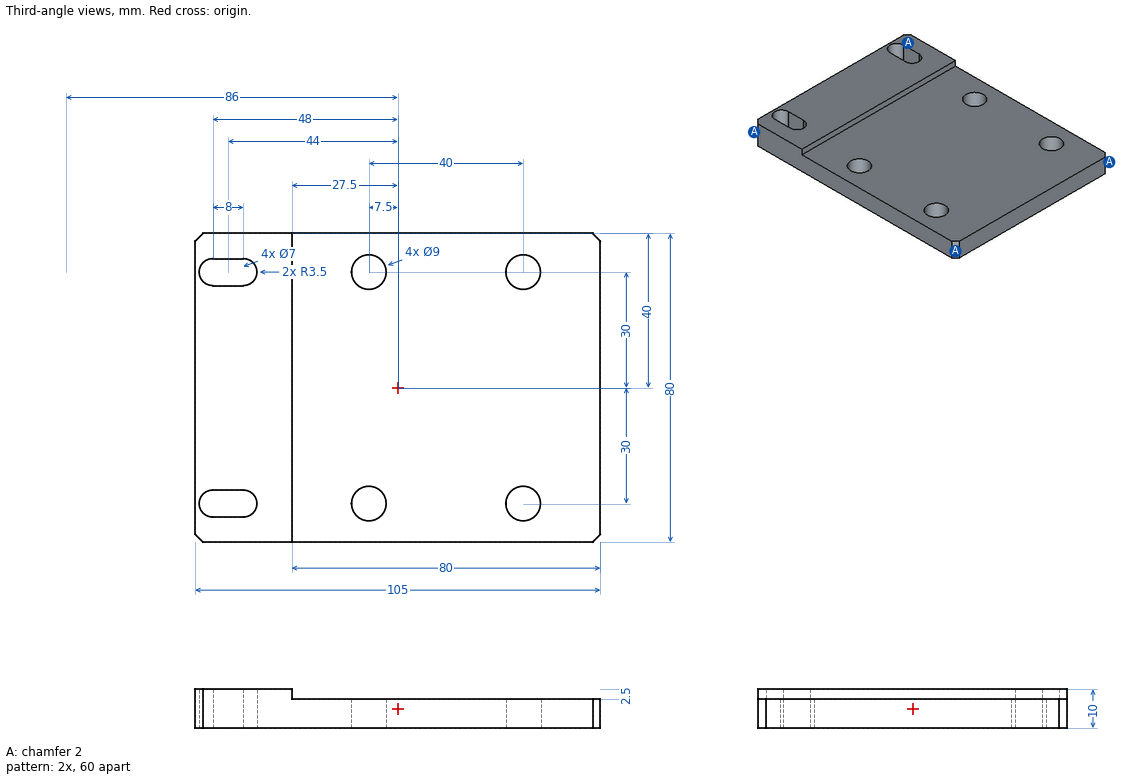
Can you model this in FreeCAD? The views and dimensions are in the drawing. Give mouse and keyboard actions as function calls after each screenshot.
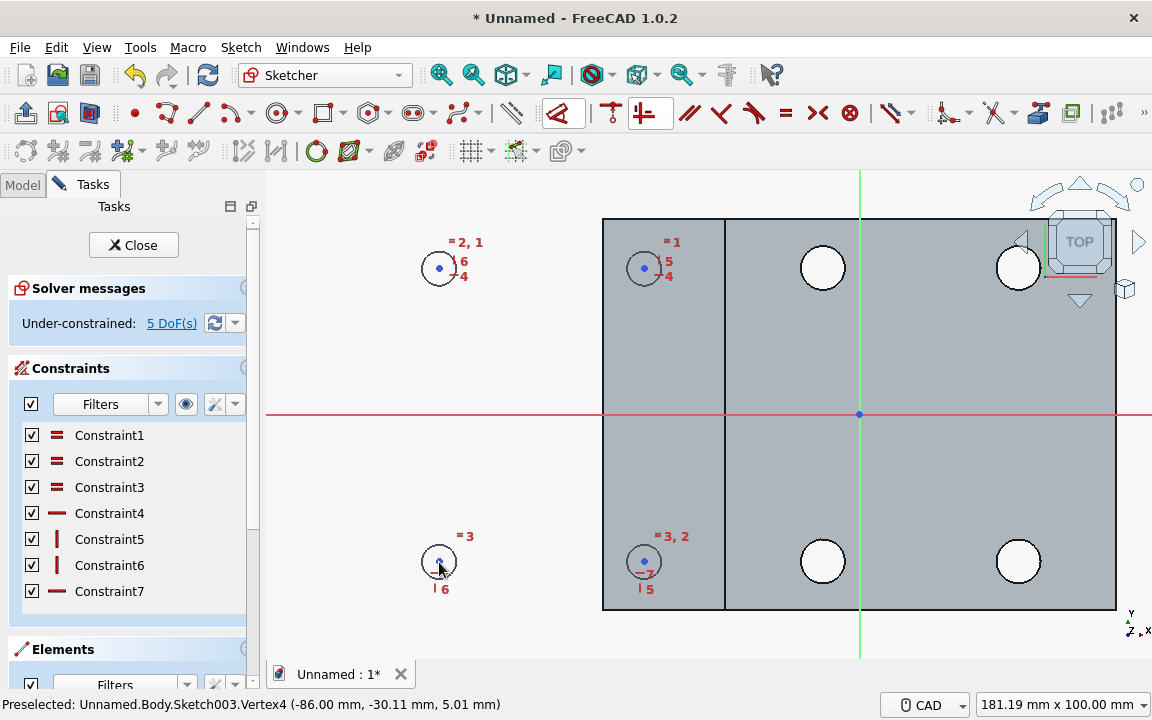
click(632, 257)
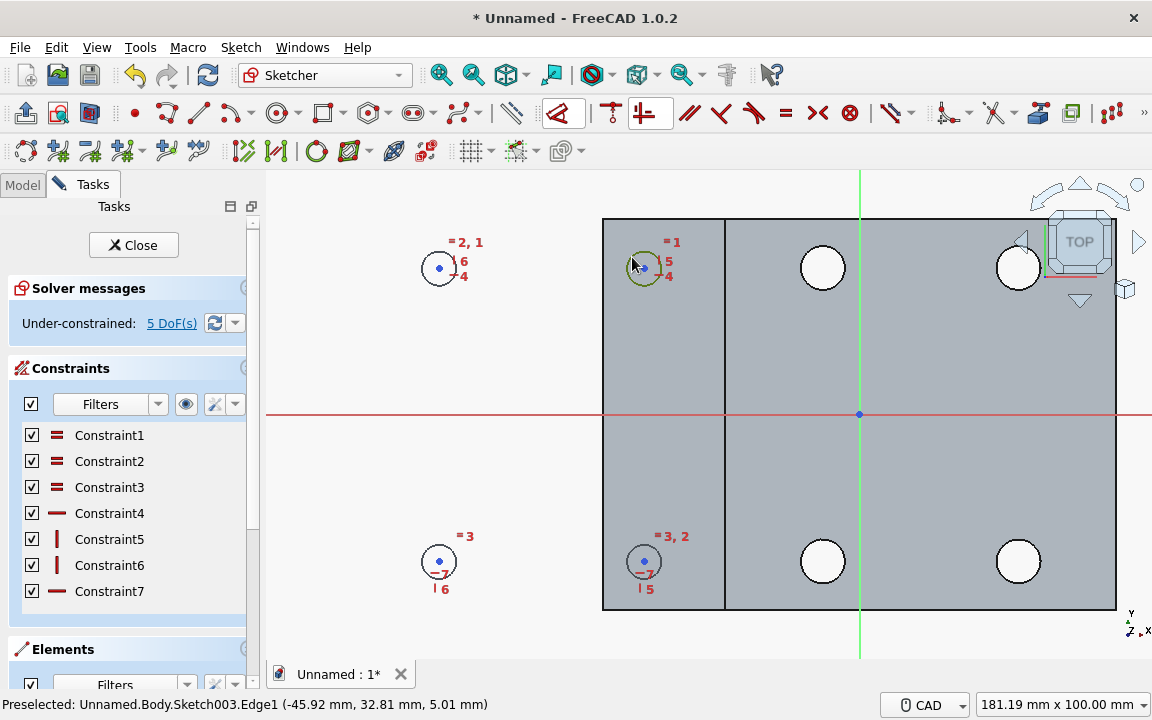
click(580, 114)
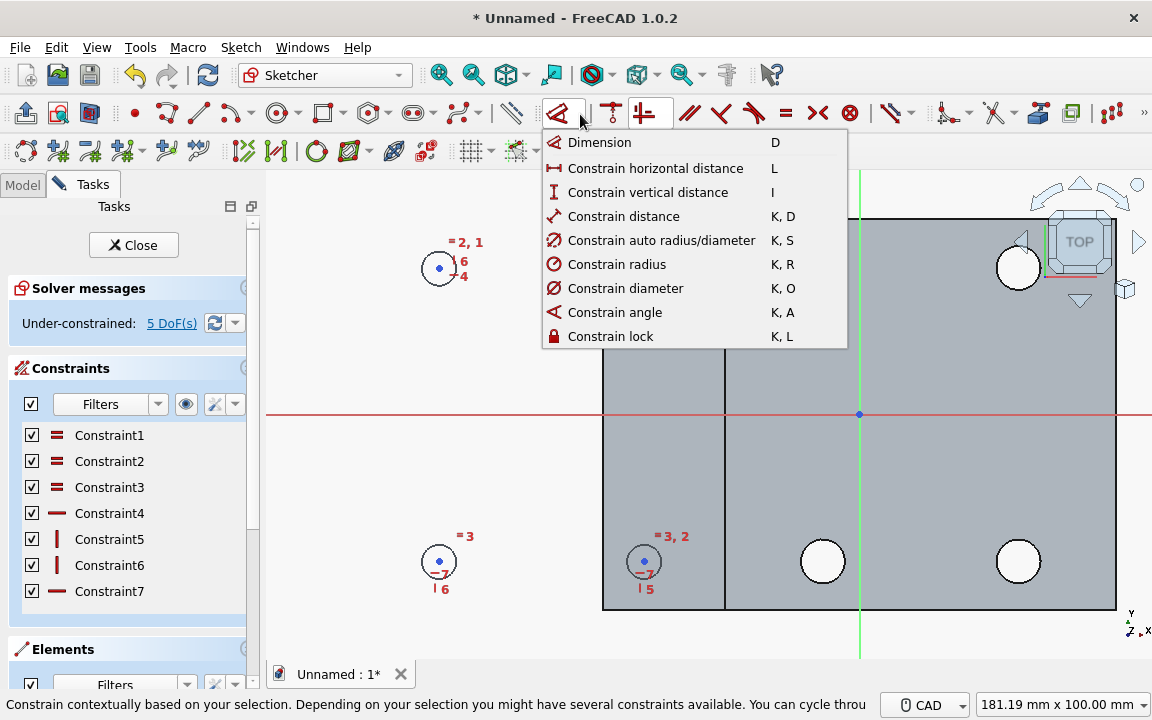
click(695, 288)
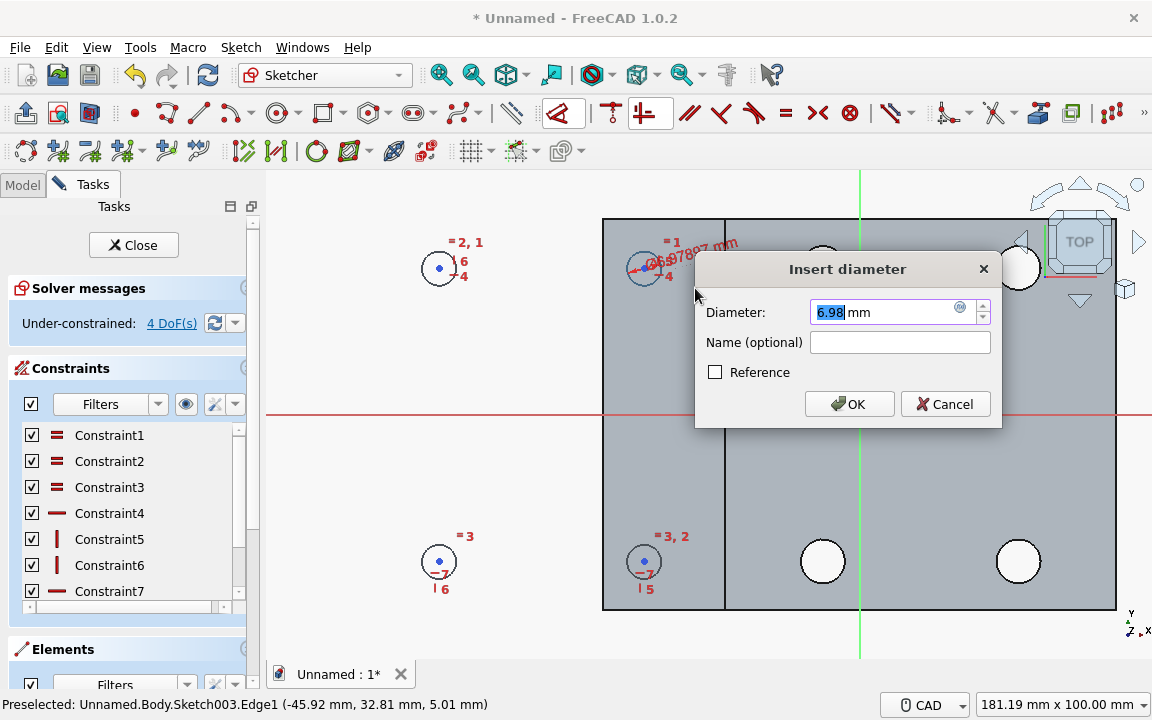
text(7)
key(Return)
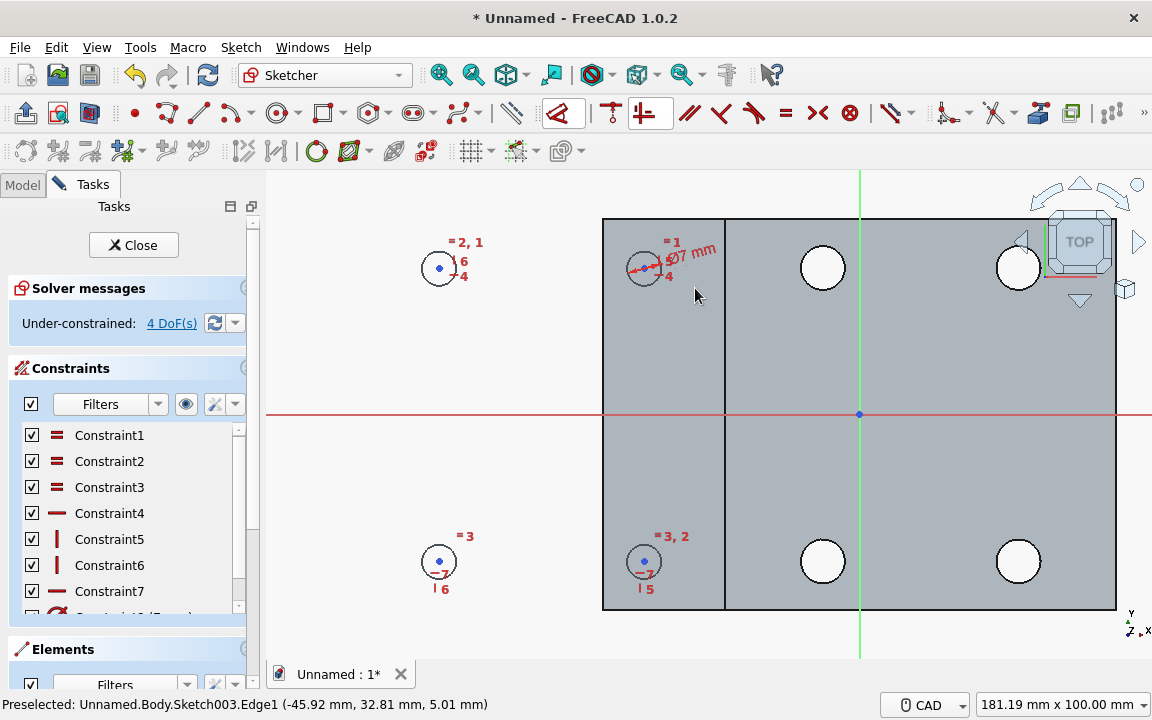
click(644, 269)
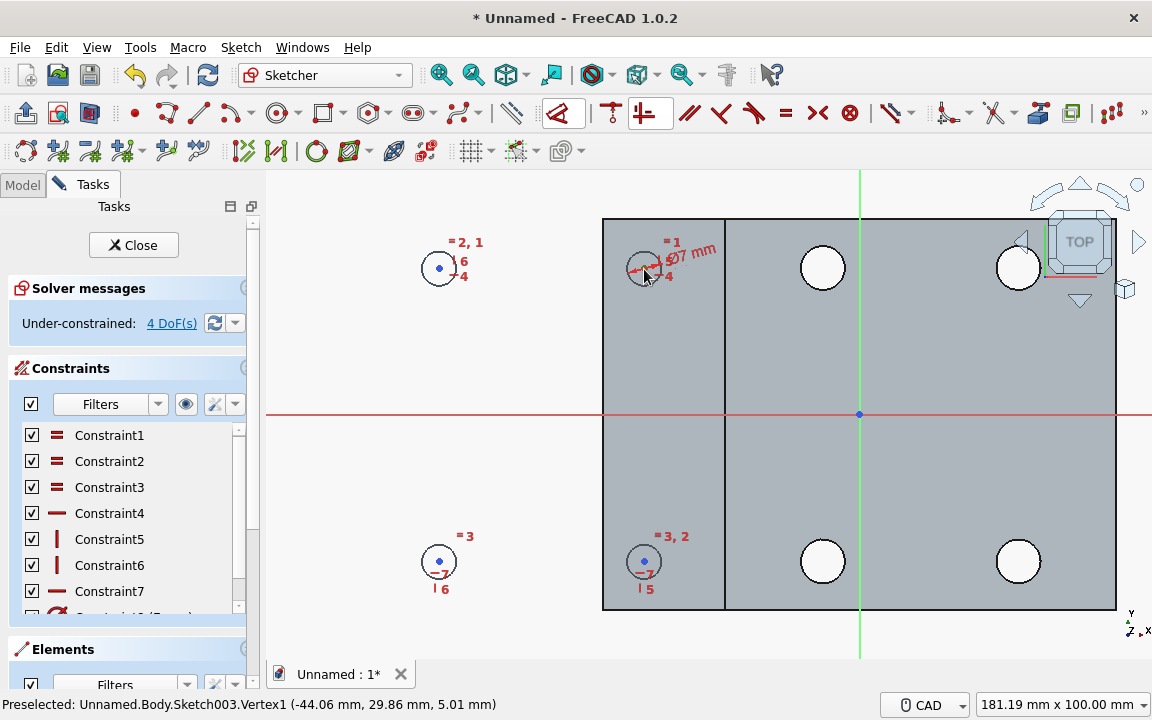
click(580, 114)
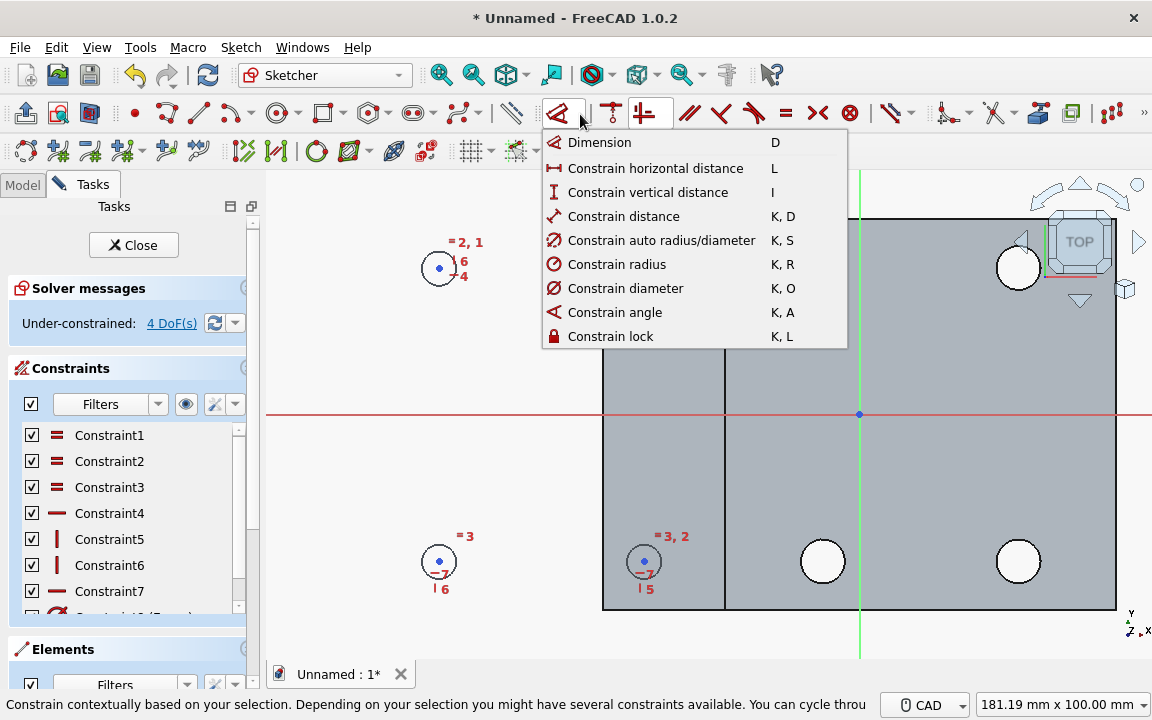
click(695, 168)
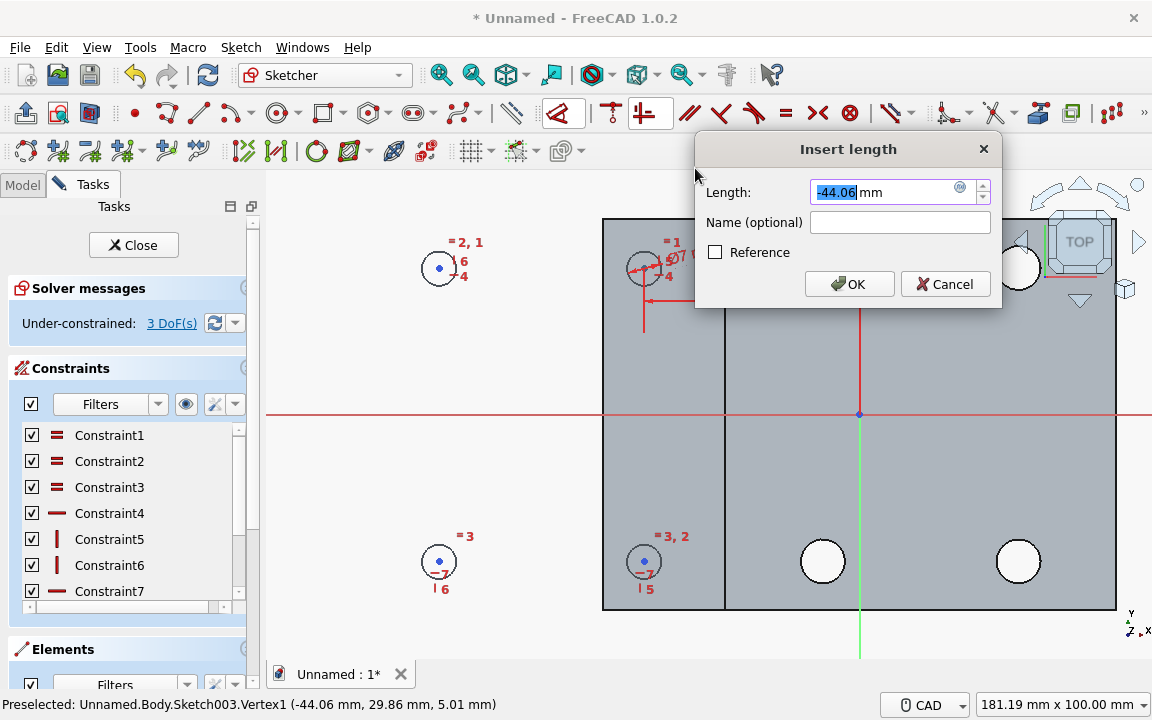
text(-44)
key(Return)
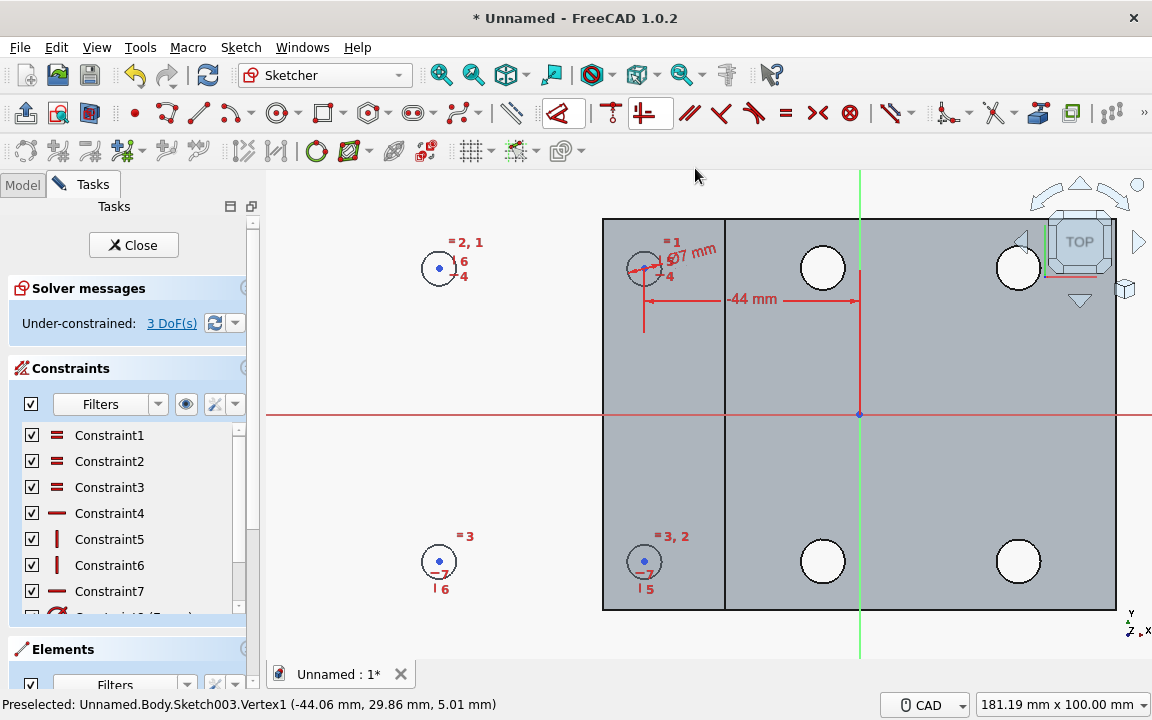
click(644, 269)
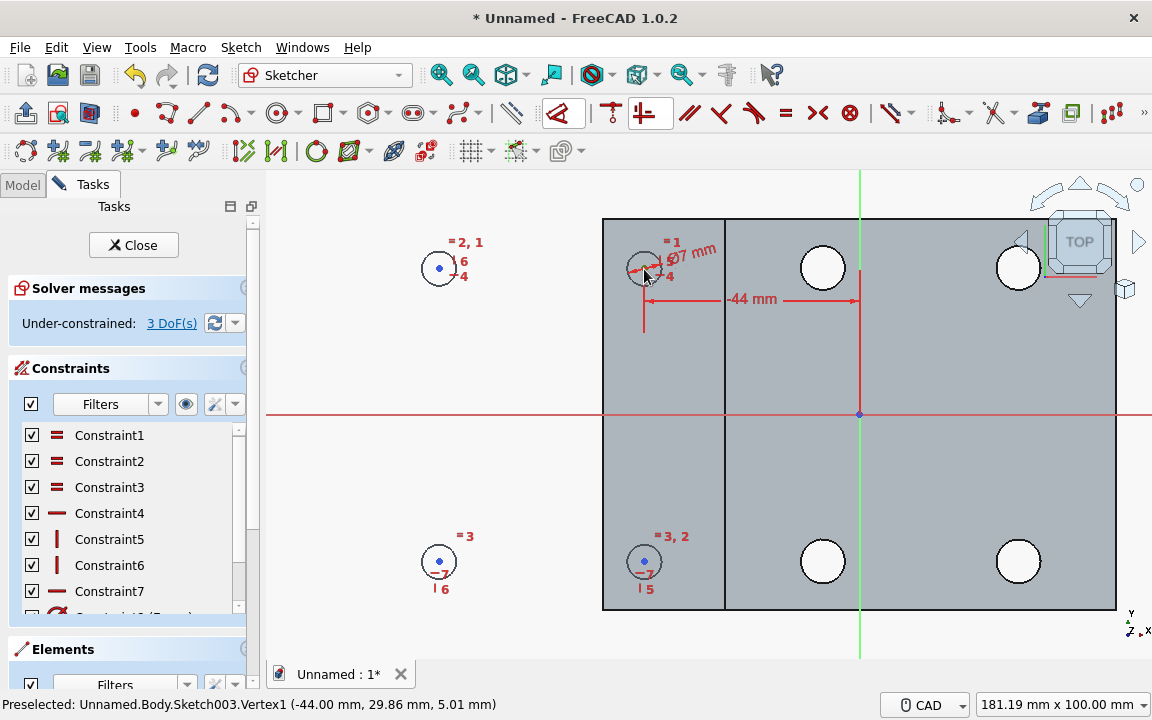
click(580, 114)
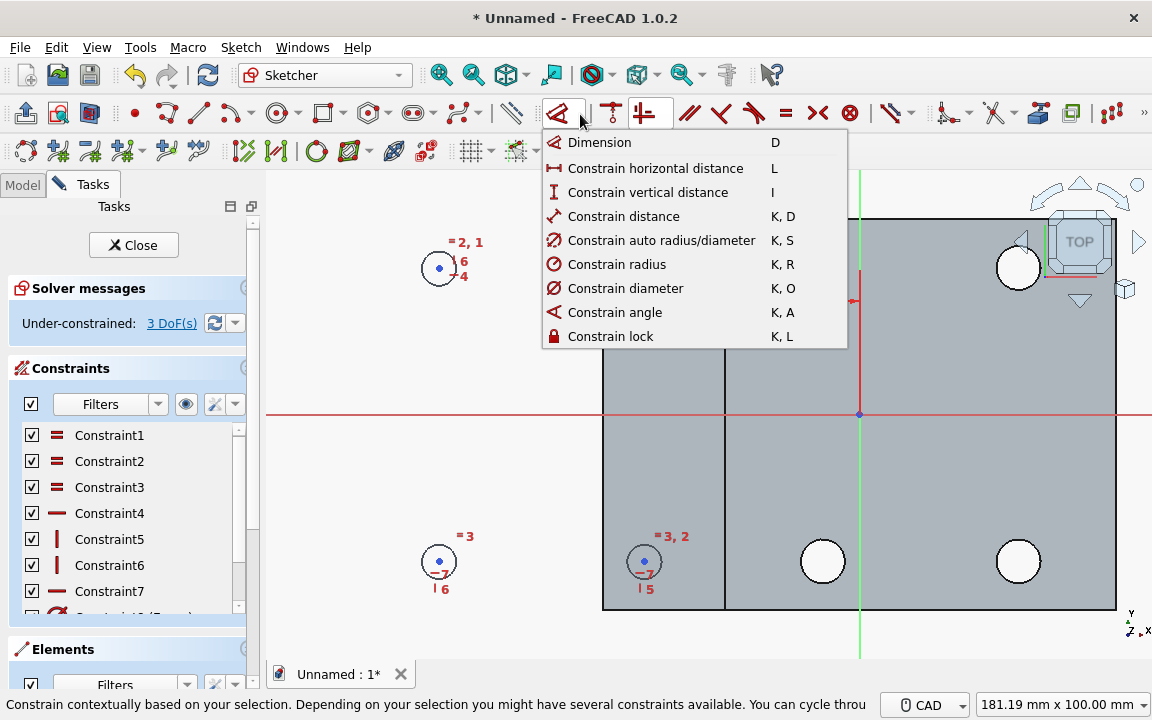
click(695, 192)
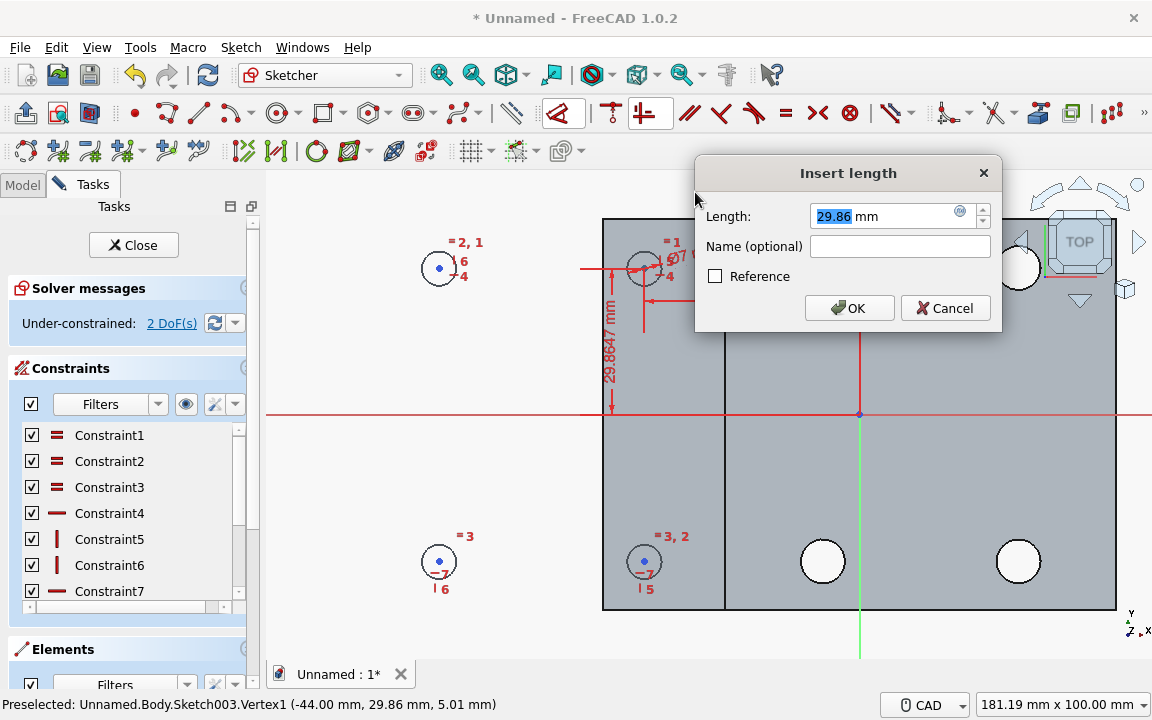
text(30)
key(Return)